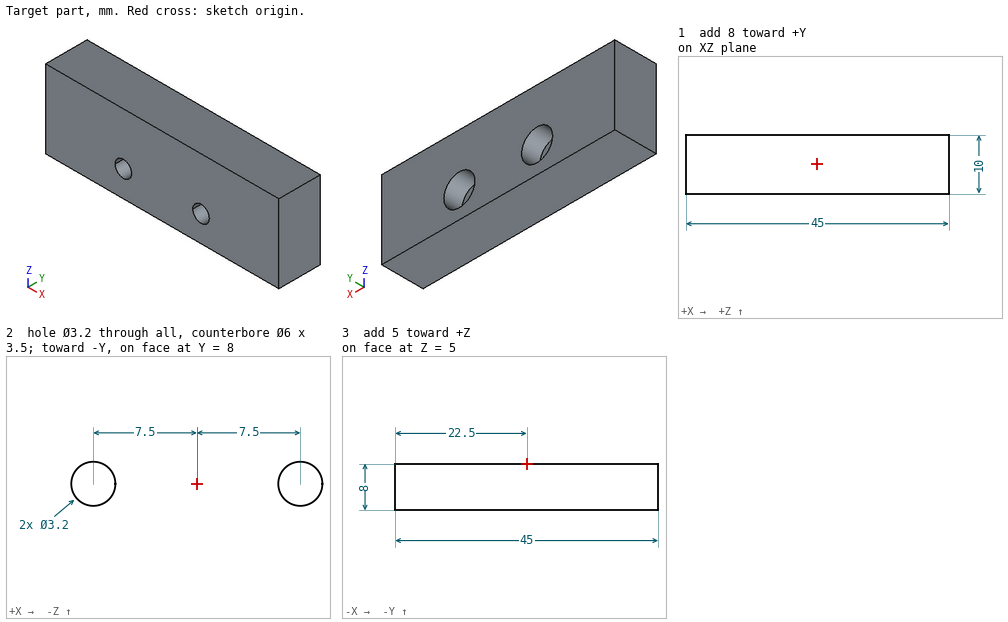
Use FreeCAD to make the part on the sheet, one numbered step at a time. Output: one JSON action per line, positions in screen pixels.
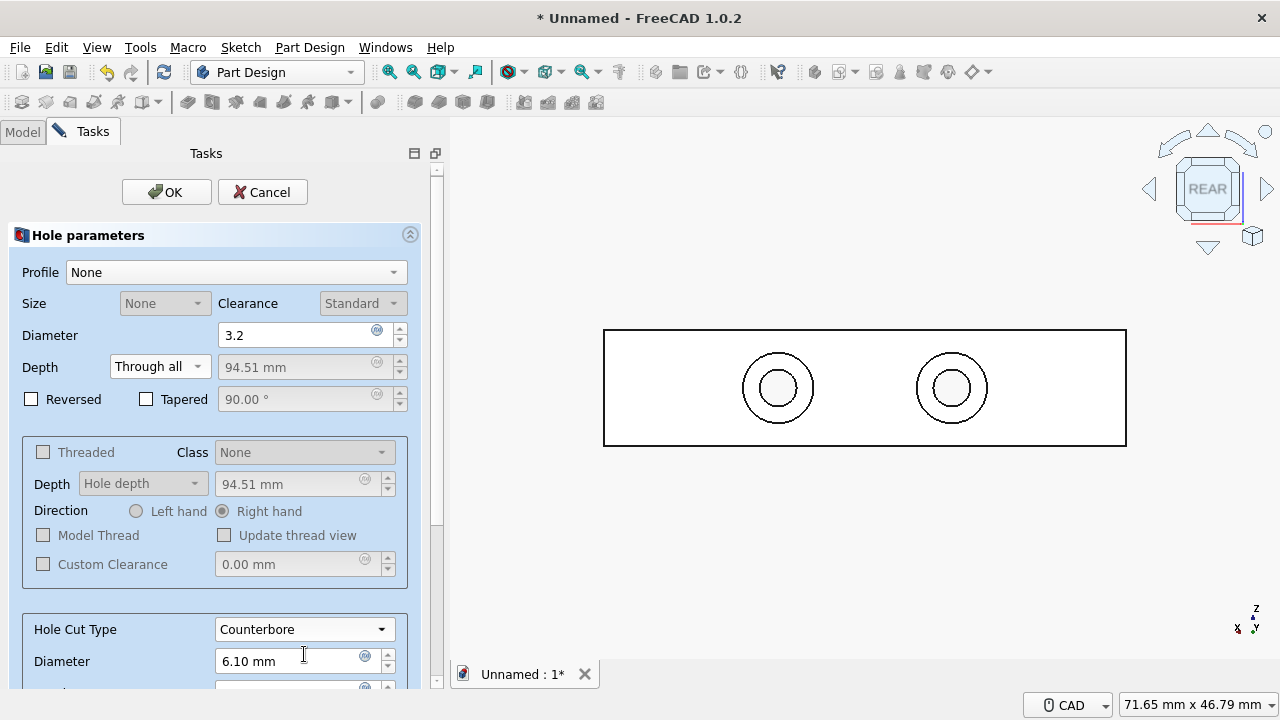
{"action": "triple_click", "coordinate": [298, 661]}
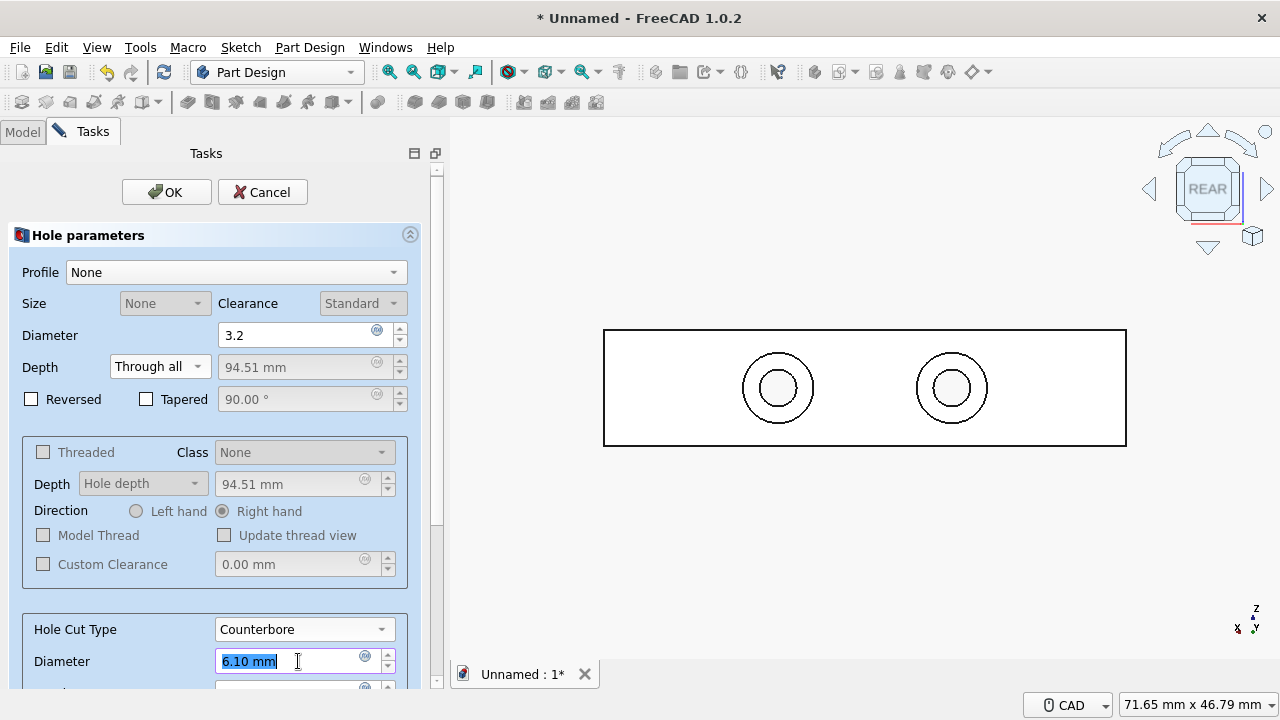
{"action": "type", "text": "6"}
{"action": "key", "text": "Tab"}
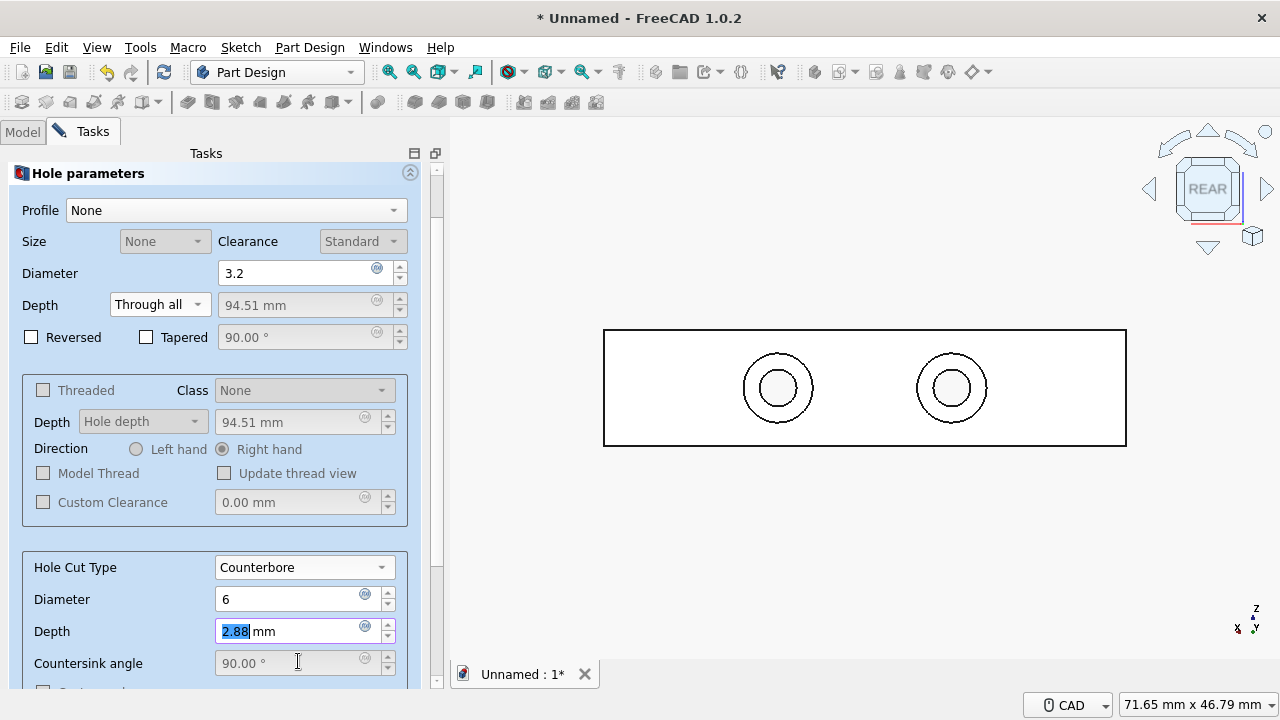
{"action": "type", "text": "3.5"}
{"action": "key", "text": "Tab"}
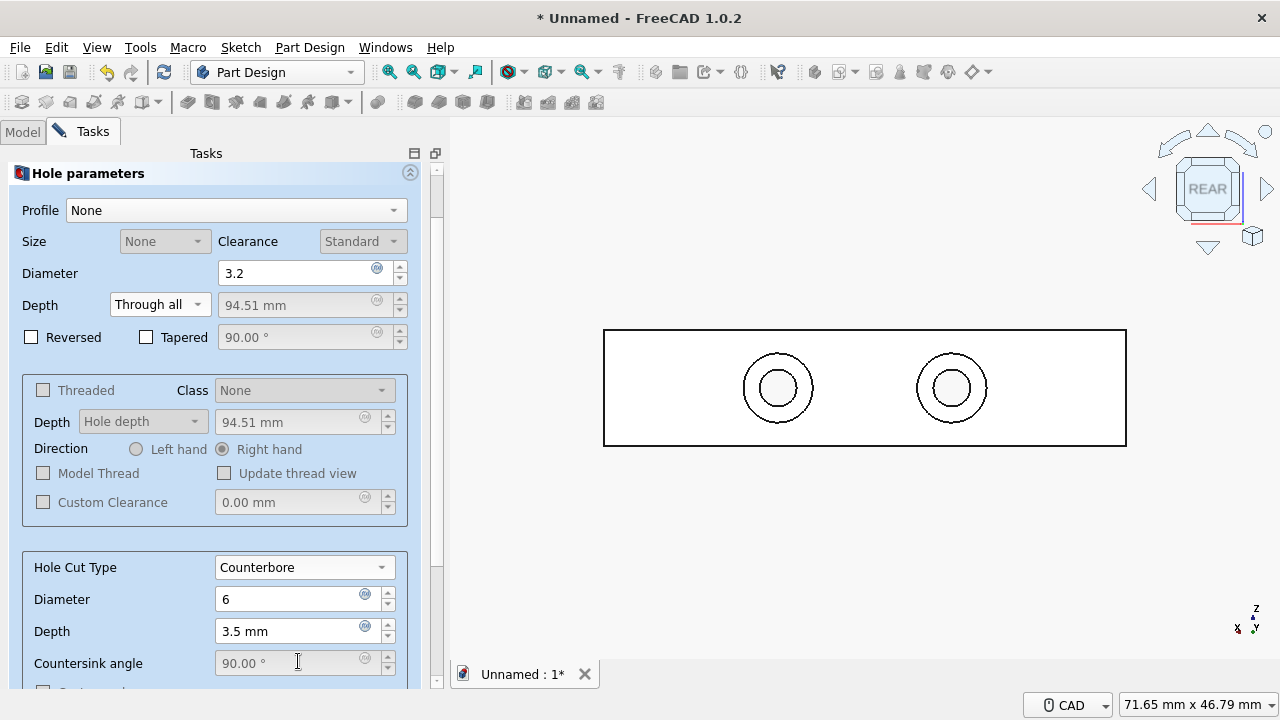
{"action": "scroll", "coordinate": [437, 426], "scroll_direction": "up", "scroll_amount": 2}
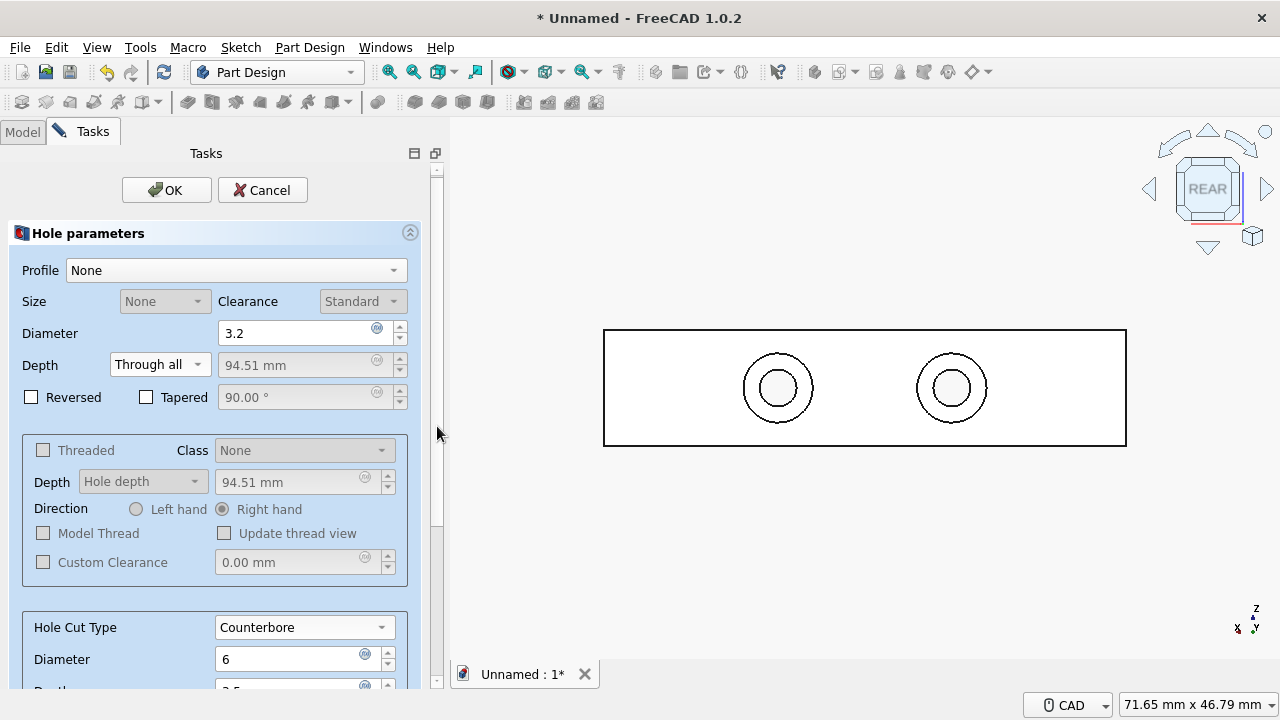
{"action": "left_click", "coordinate": [167, 192]}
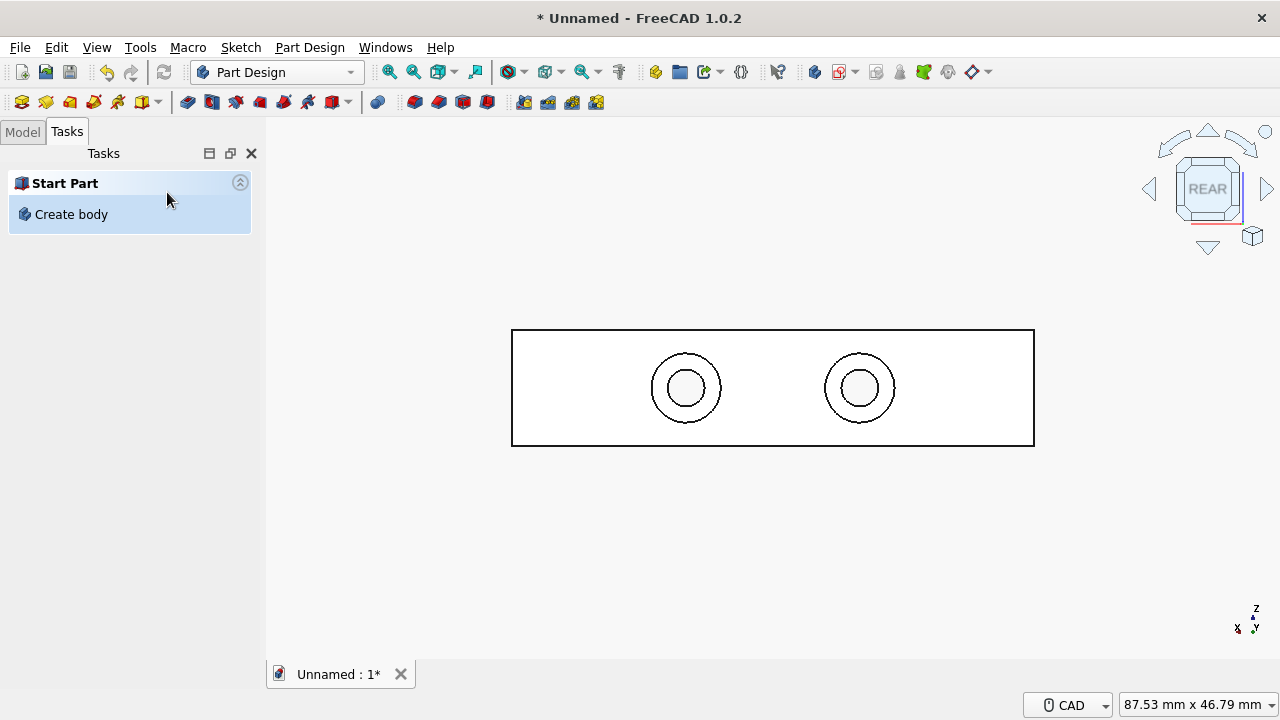
{"action": "key", "text": "0"}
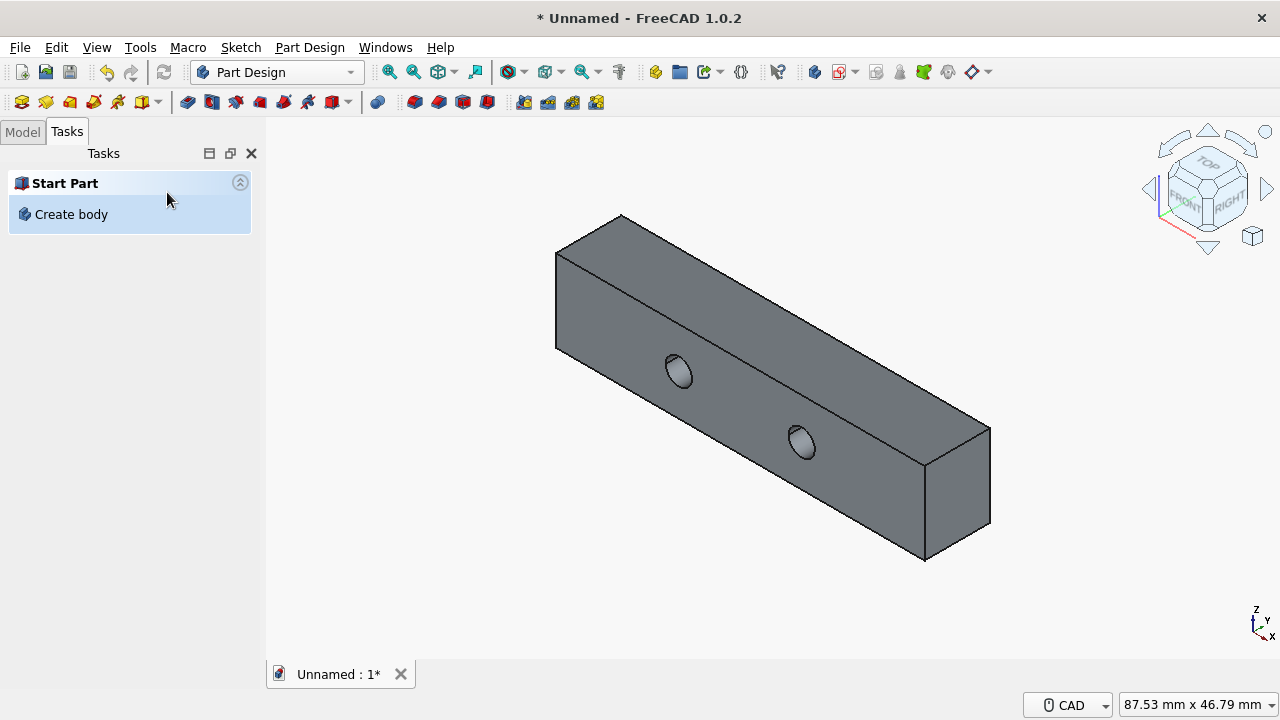
{"action": "left_click", "coordinate": [878, 401]}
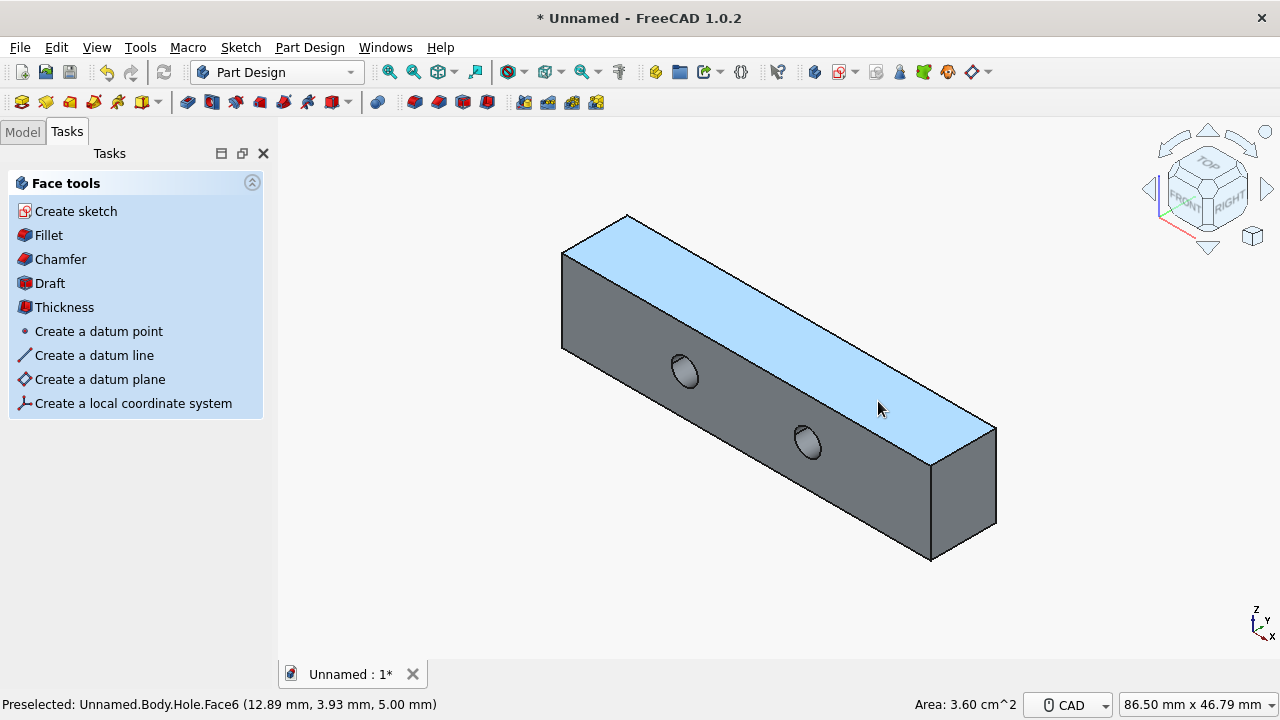
{"action": "left_click", "coordinate": [840, 72]}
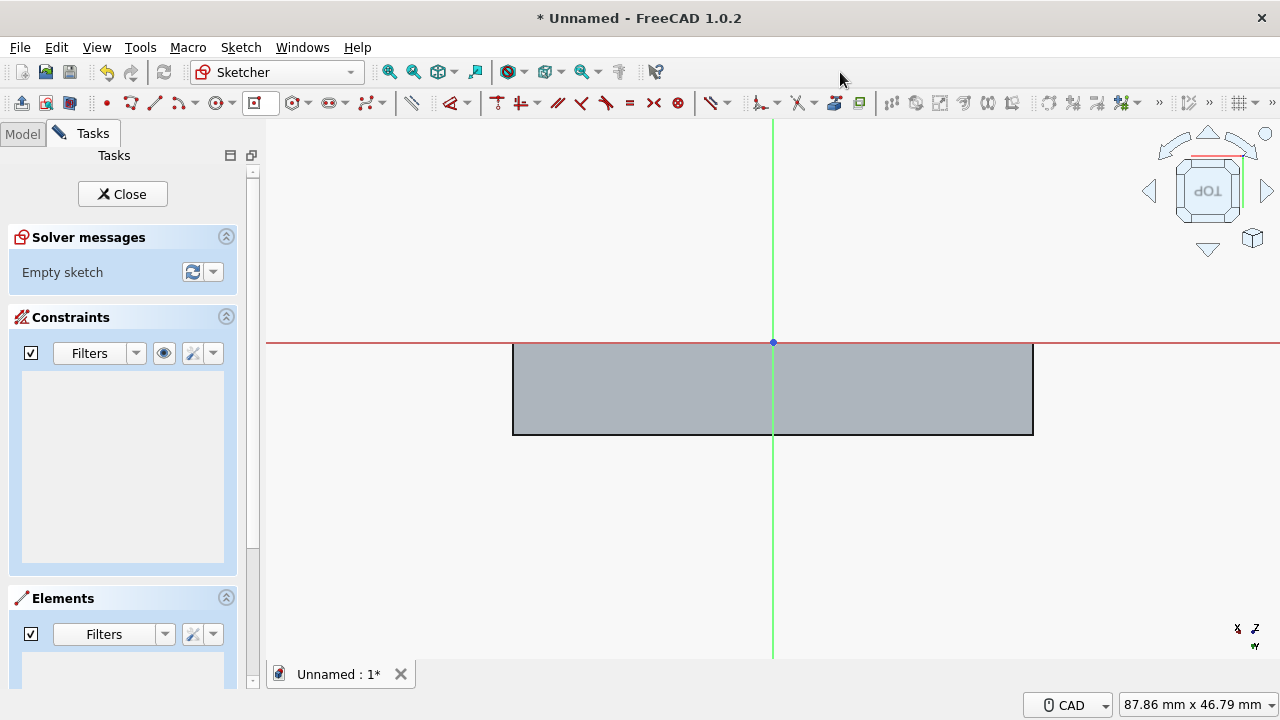
{"action": "left_click", "coordinate": [274, 104]}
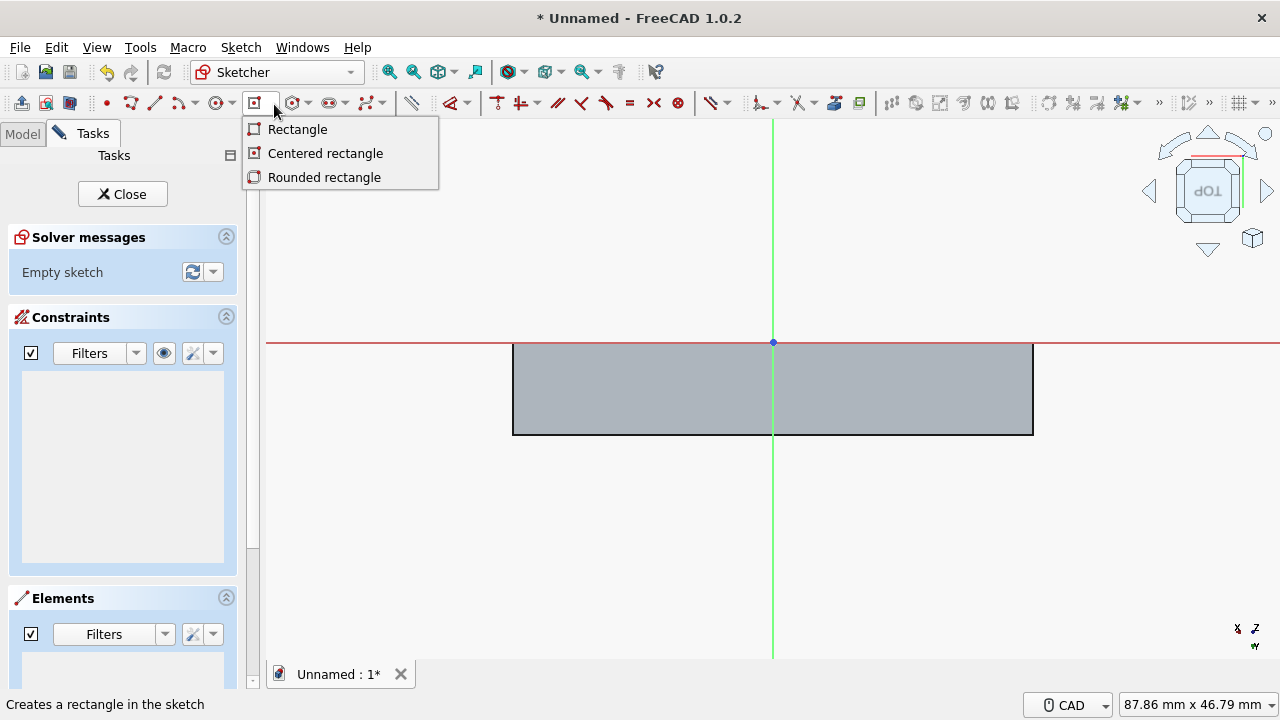
{"action": "left_click", "coordinate": [340, 129]}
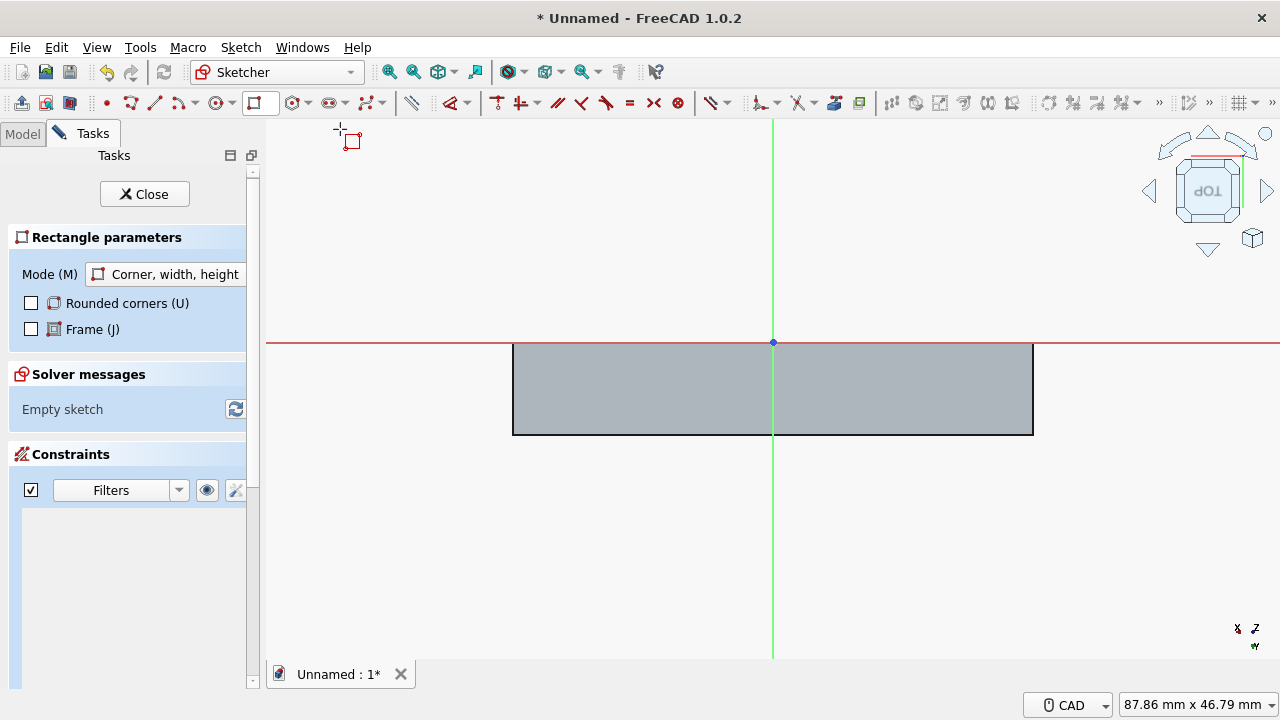
{"action": "left_click", "coordinate": [513, 343]}
{"action": "left_click", "coordinate": [1033, 435]}
{"action": "key", "text": "Escape"}